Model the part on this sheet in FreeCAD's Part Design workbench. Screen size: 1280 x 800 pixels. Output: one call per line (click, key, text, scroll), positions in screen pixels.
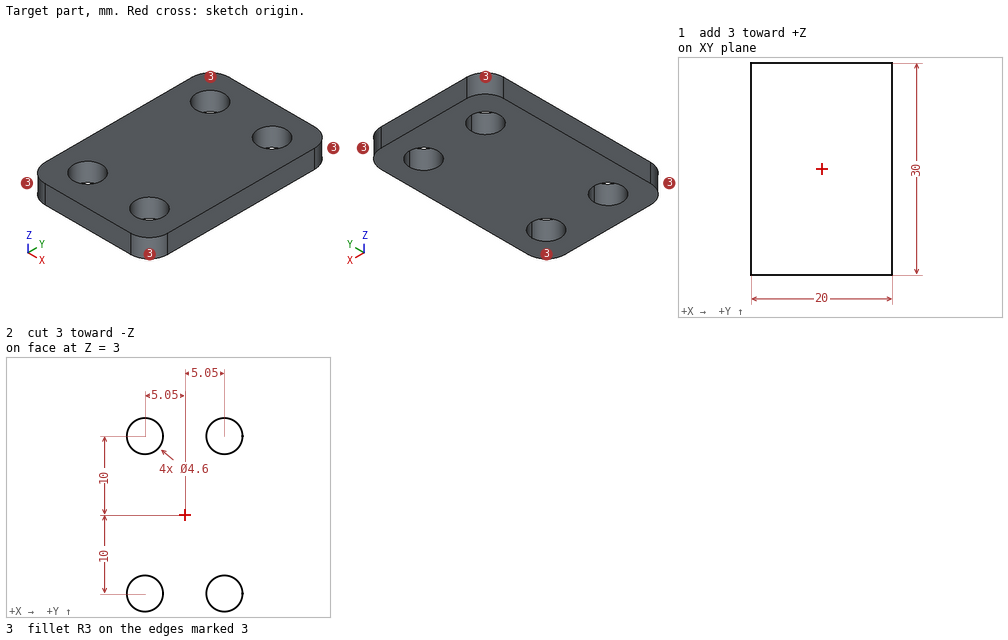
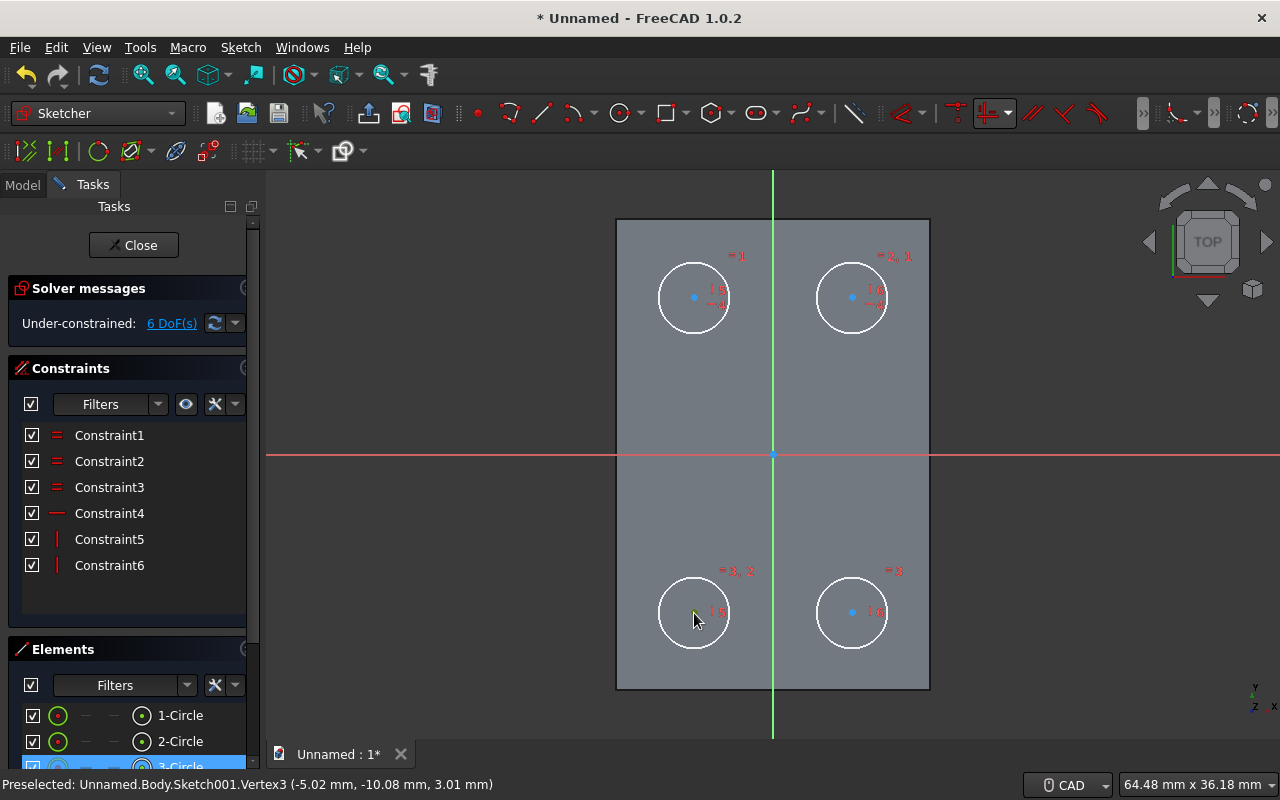
click(852, 613)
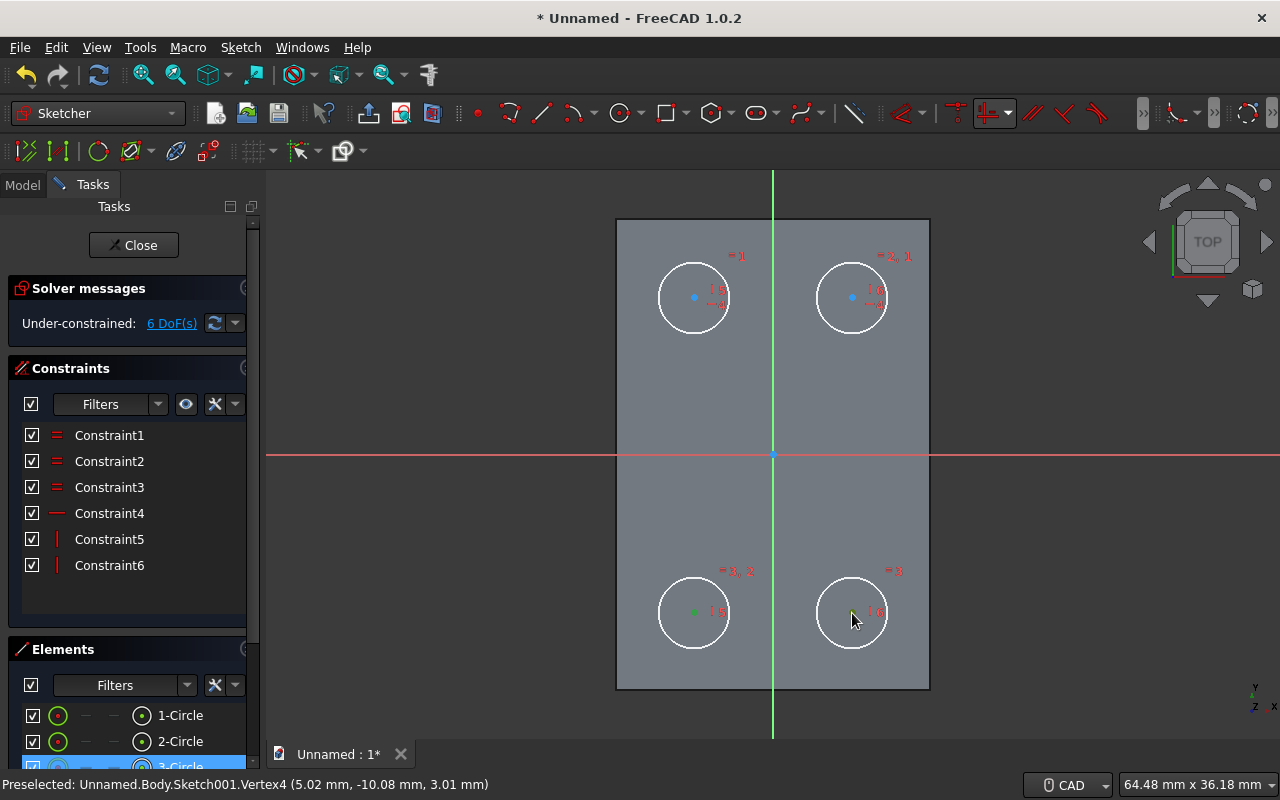
key(h)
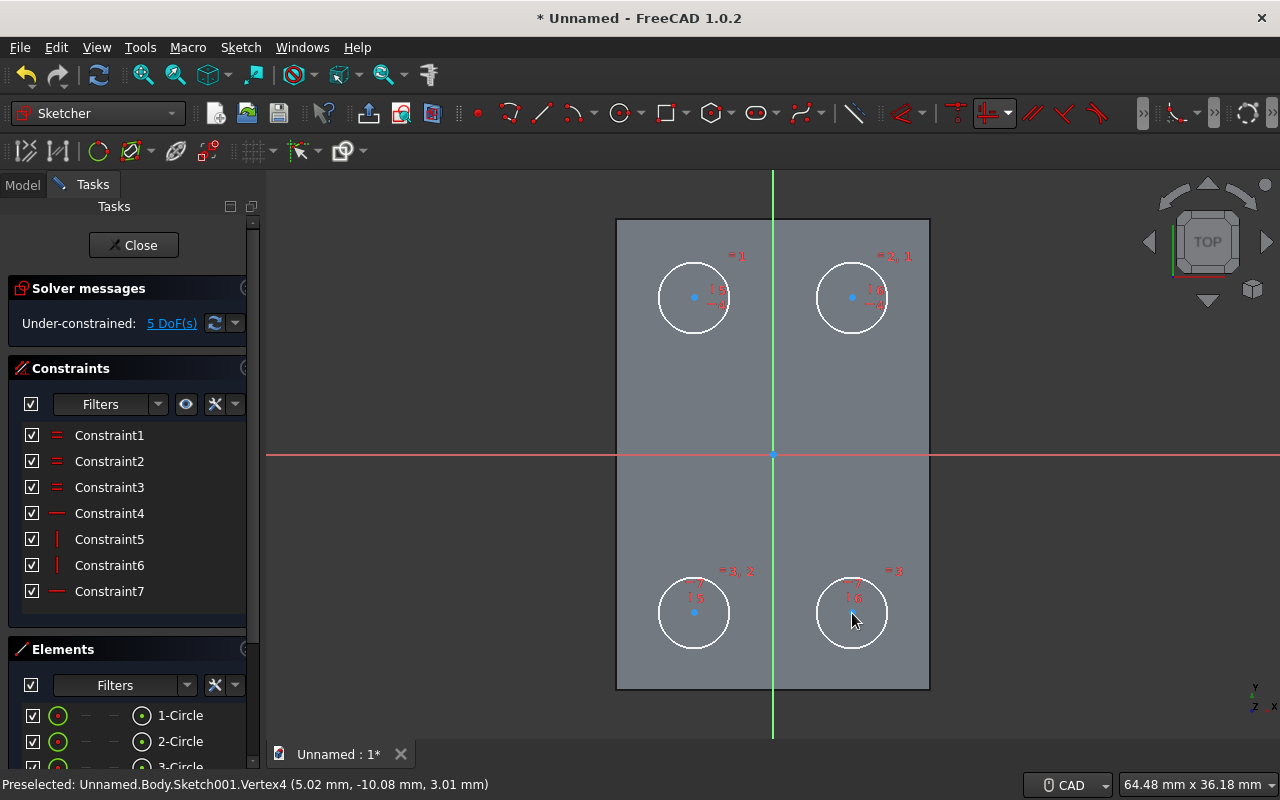
click(902, 114)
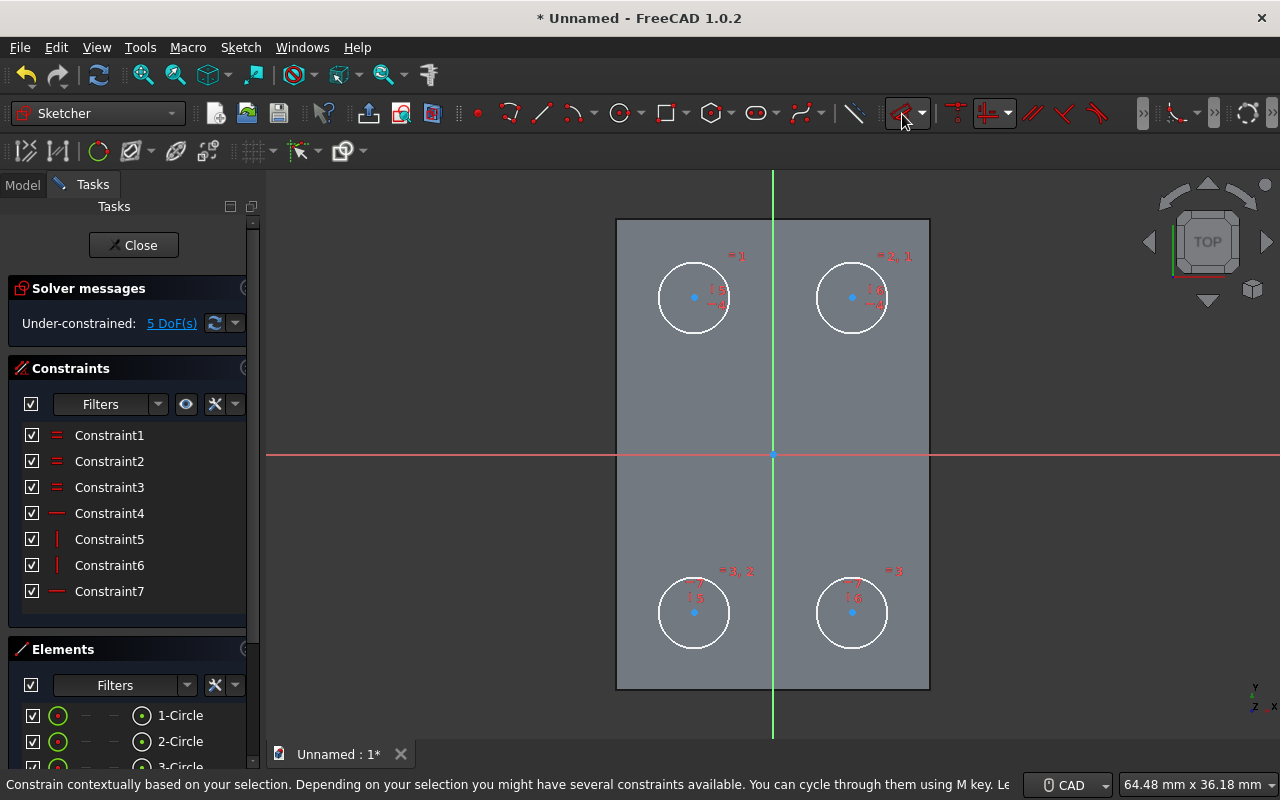
click(719, 273)
click(742, 250)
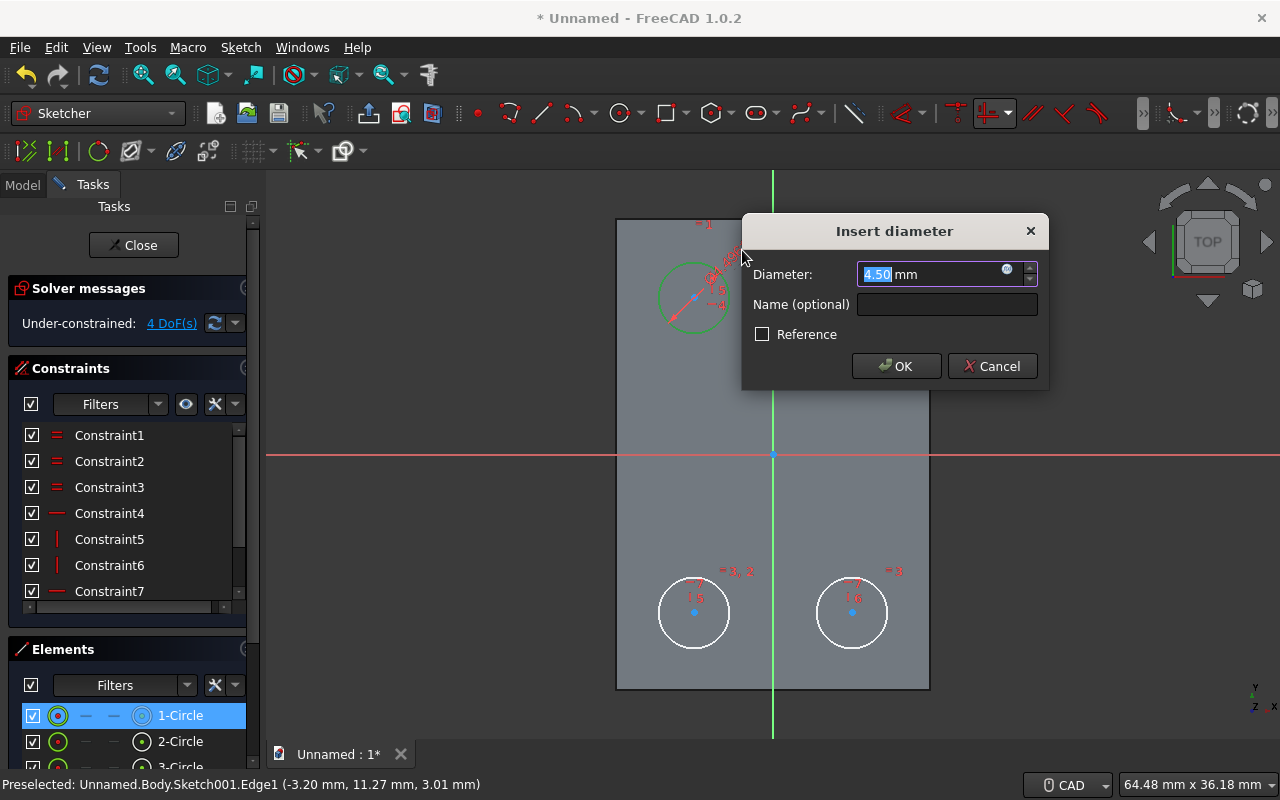
text(4.6)
key(Return)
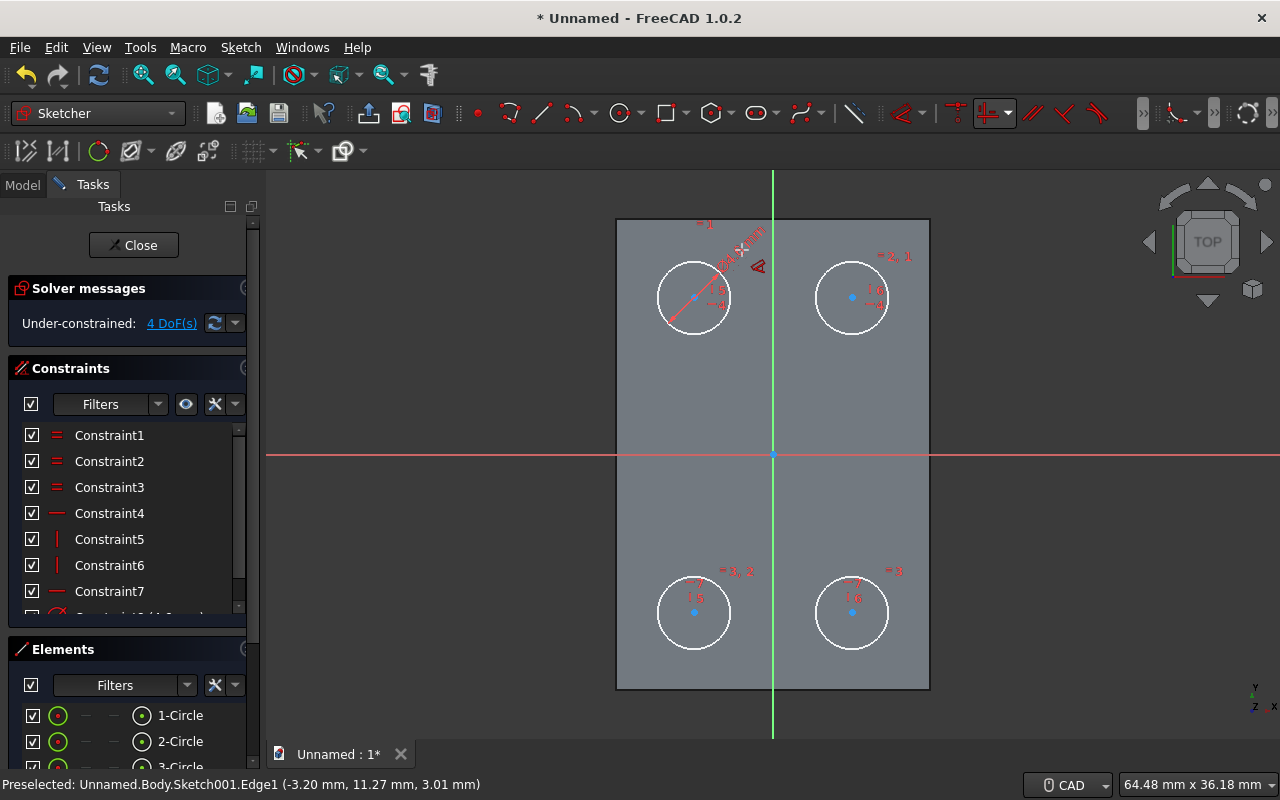
click(694, 298)
click(660, 376)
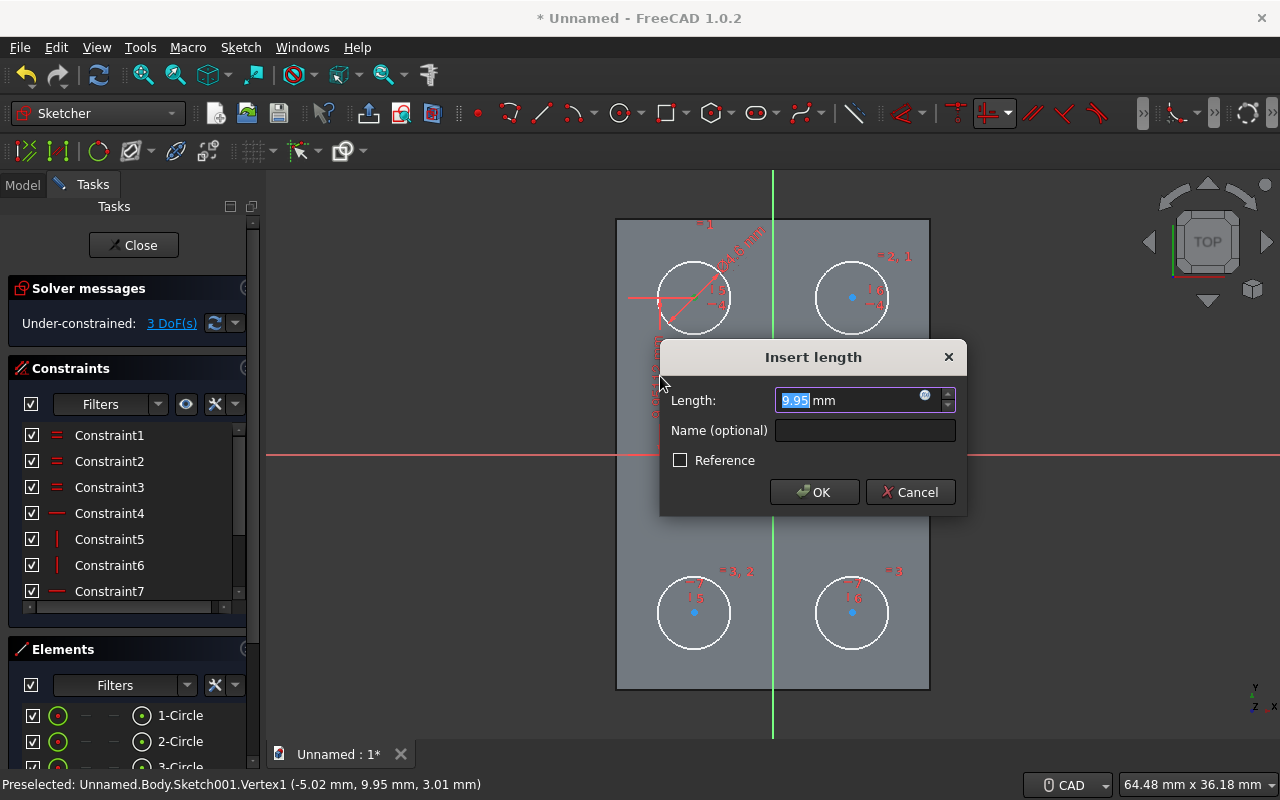
text(10)
key(Return)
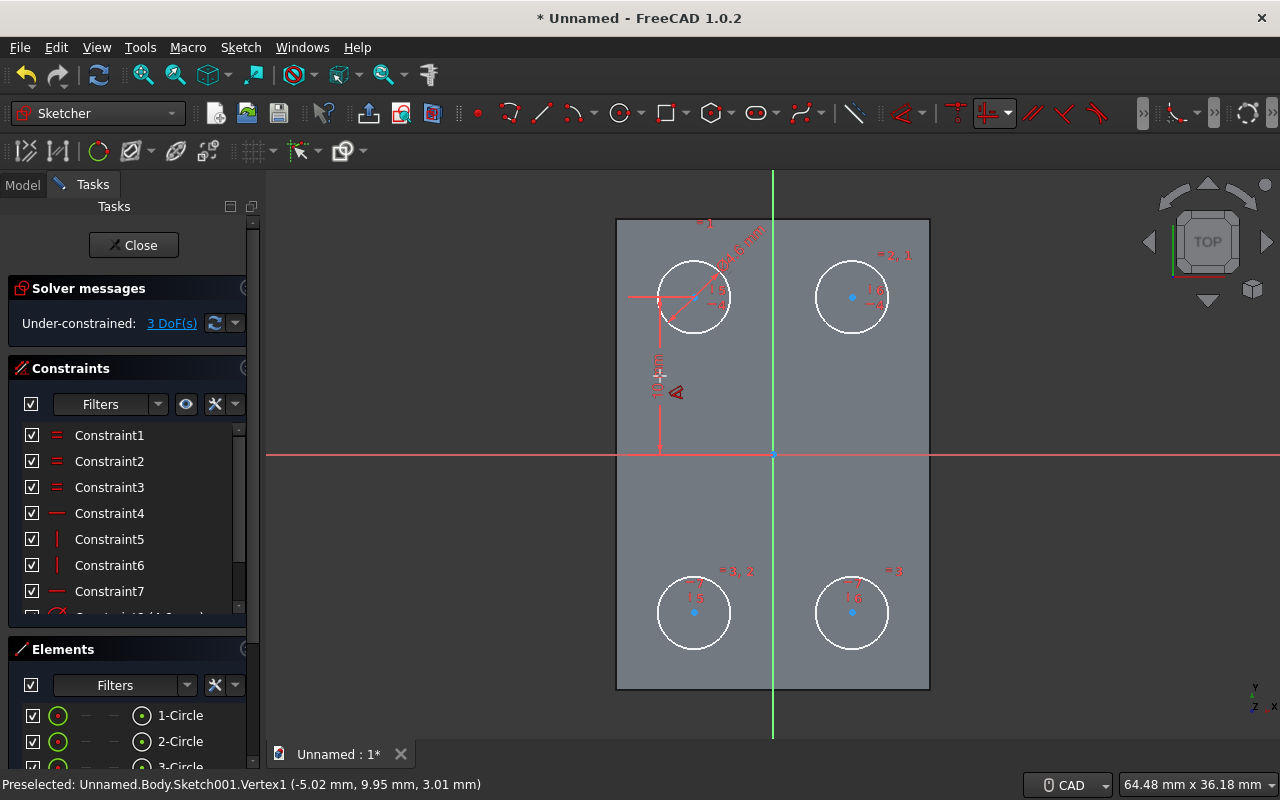
click(694, 613)
click(660, 534)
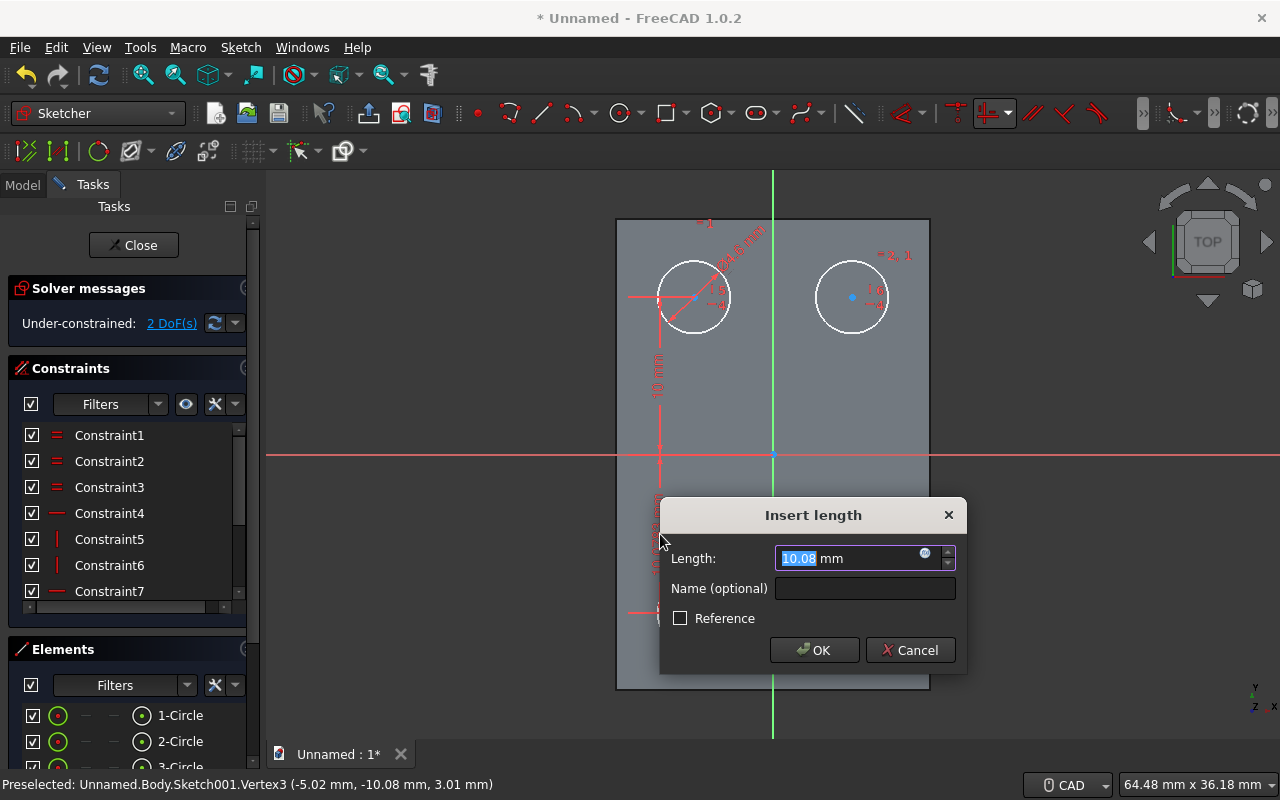
text(10)
key(Return)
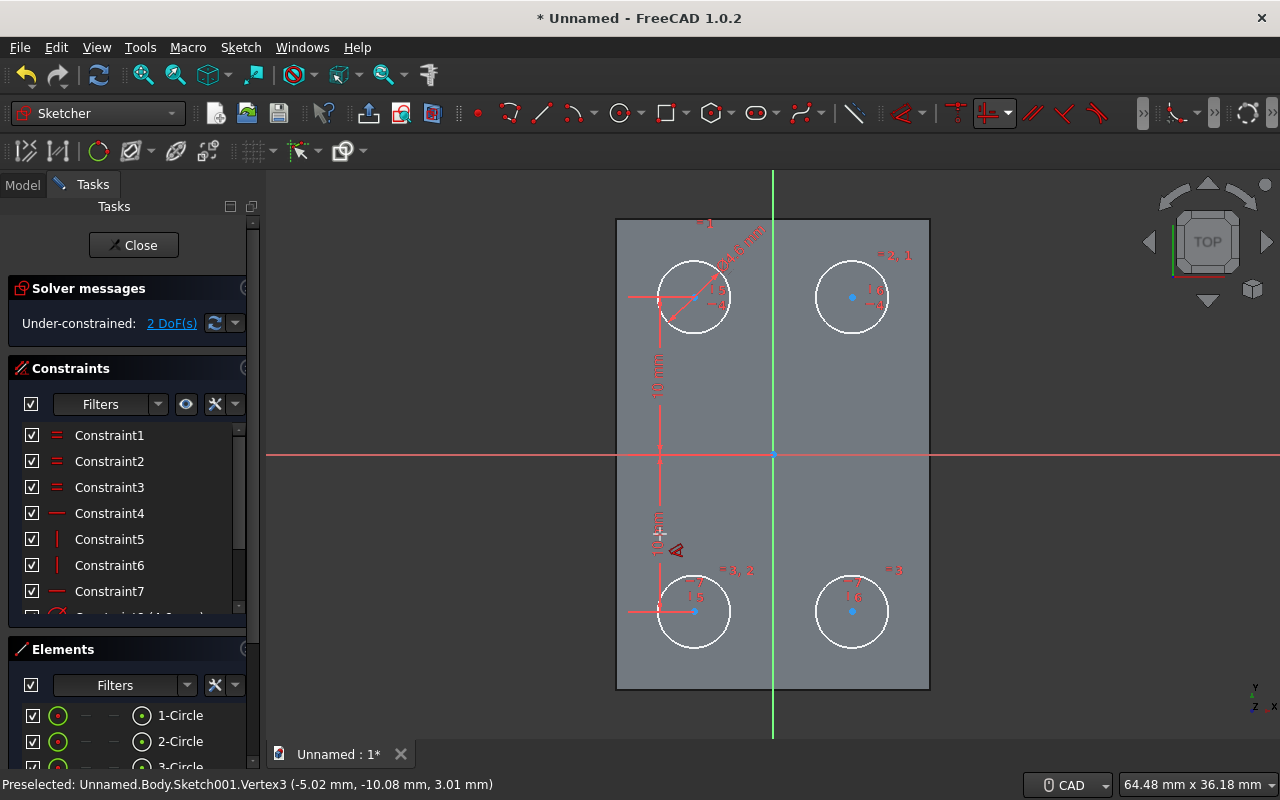
click(694, 297)
click(734, 488)